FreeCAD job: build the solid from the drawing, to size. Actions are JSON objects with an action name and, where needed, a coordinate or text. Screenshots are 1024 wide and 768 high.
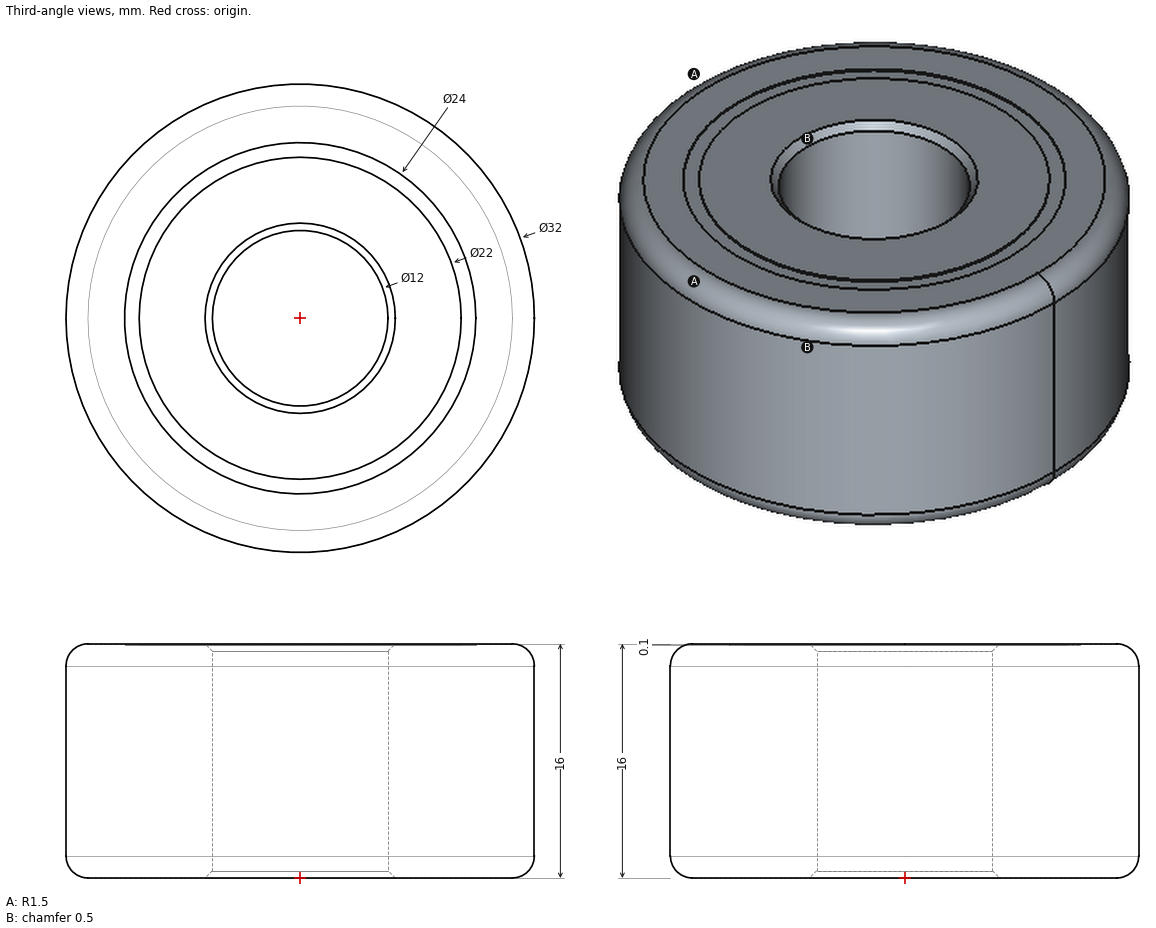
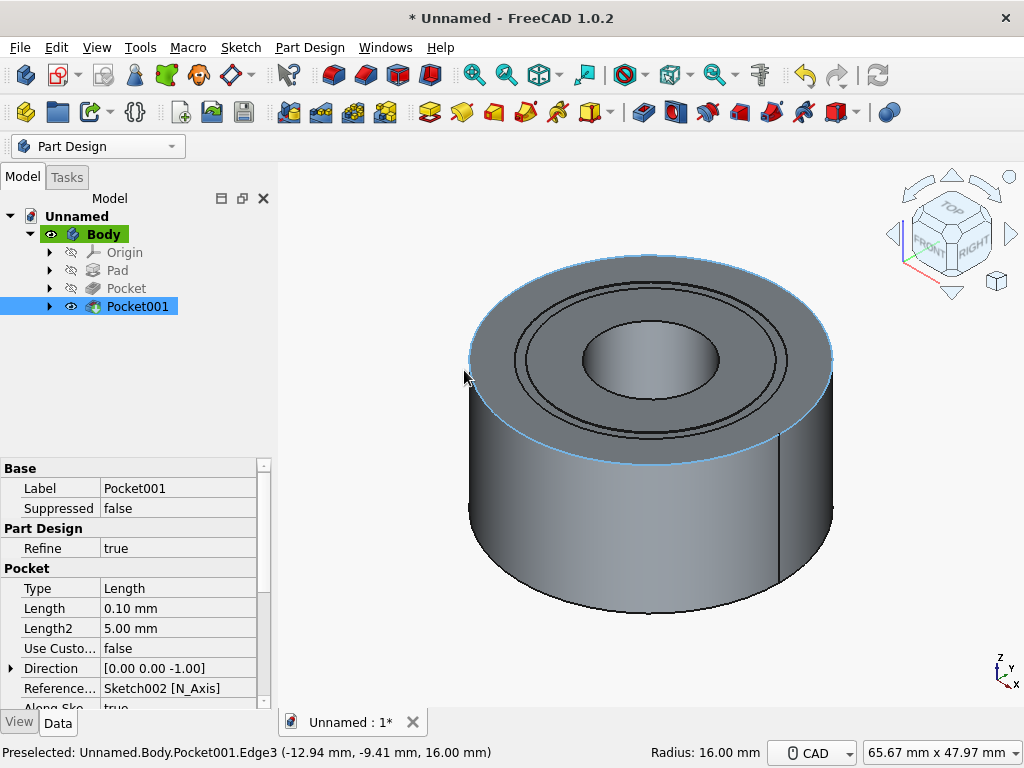
{"action": "key", "text": "2"}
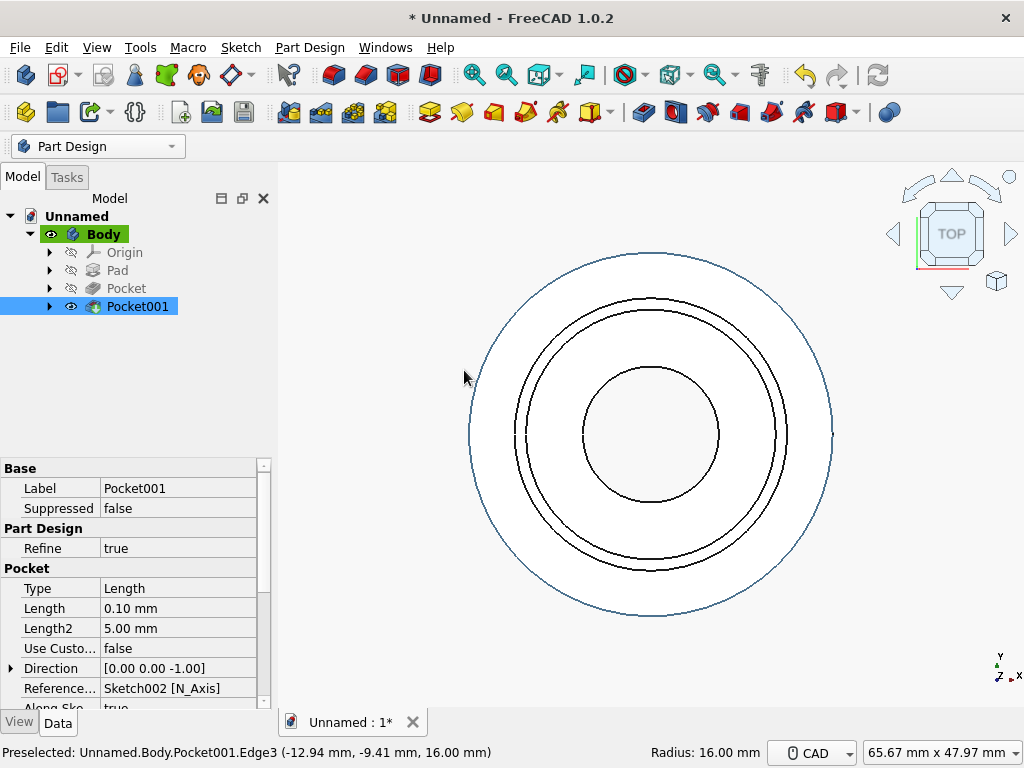
{"action": "key", "text": "1"}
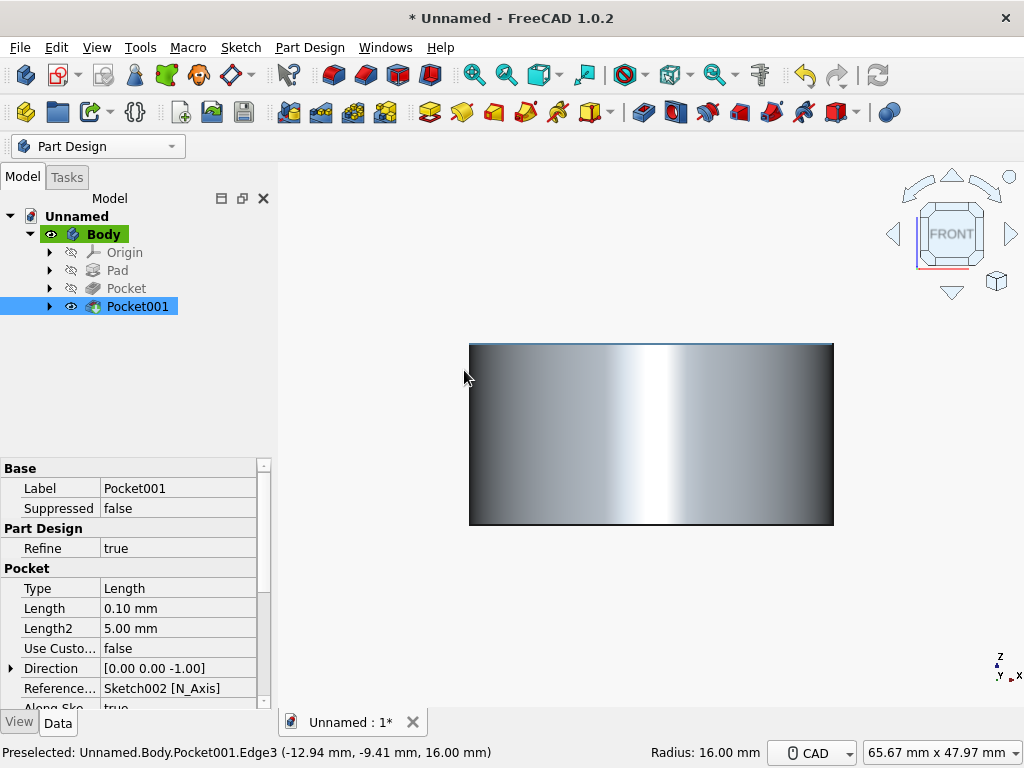
{"action": "left_click", "coordinate": [504, 524], "text": "ctrl"}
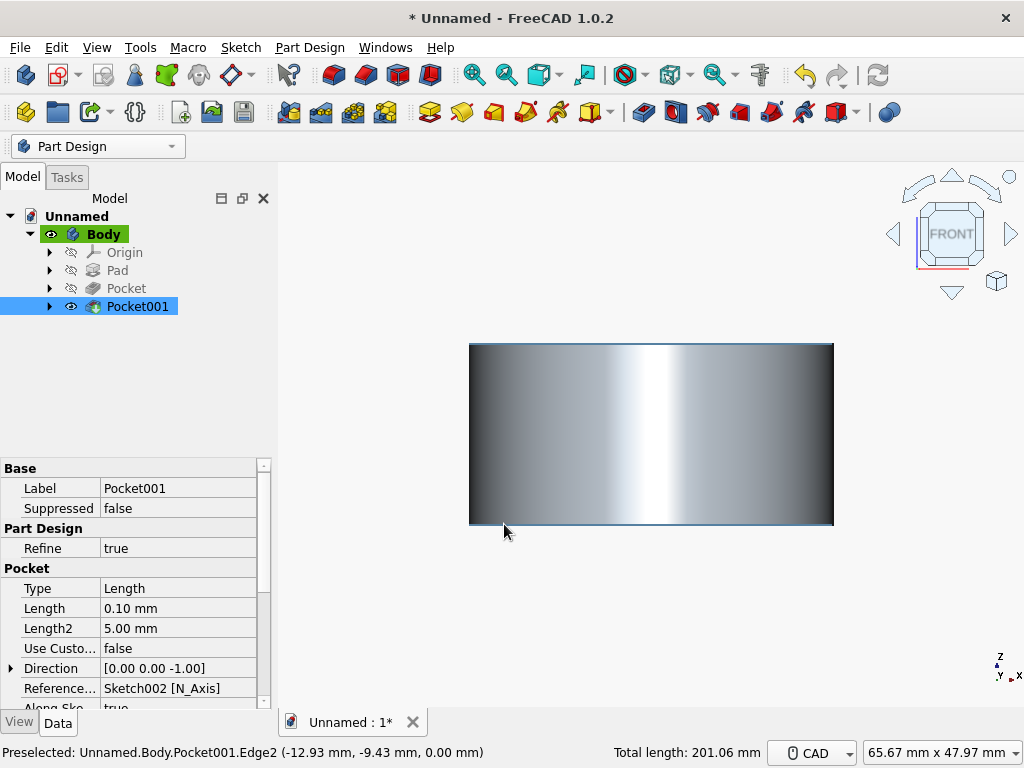
{"action": "left_click", "coordinate": [334, 76]}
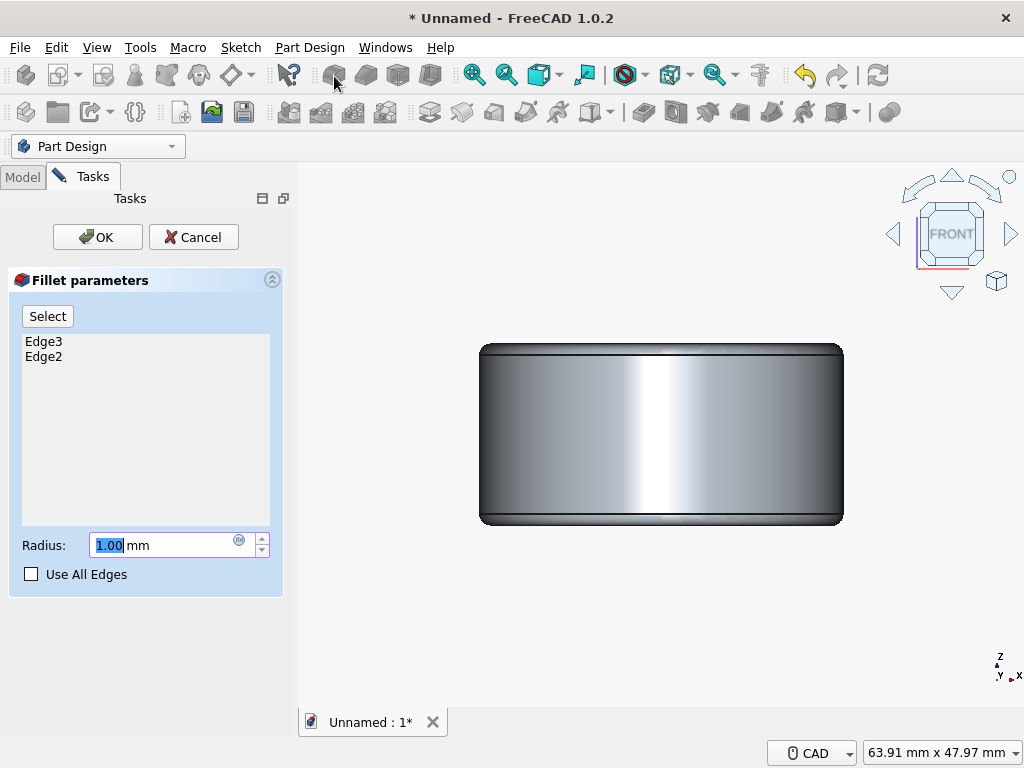
{"action": "type", "text": "1.5"}
{"action": "key", "text": "Tab"}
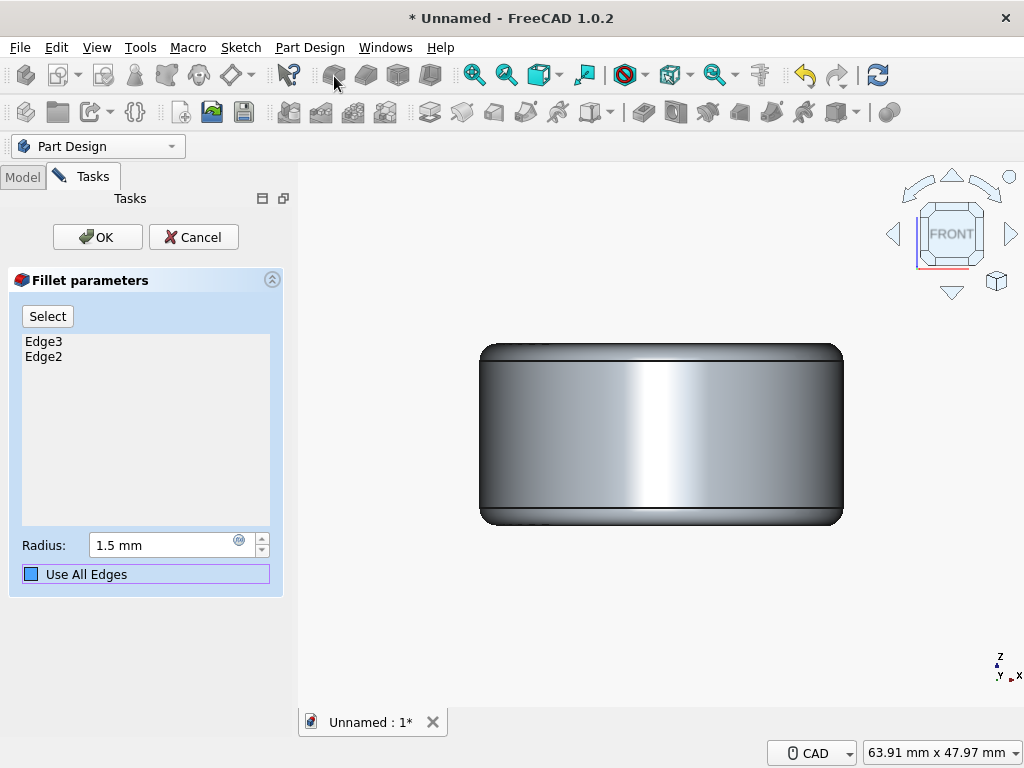
{"action": "left_click", "coordinate": [98, 237]}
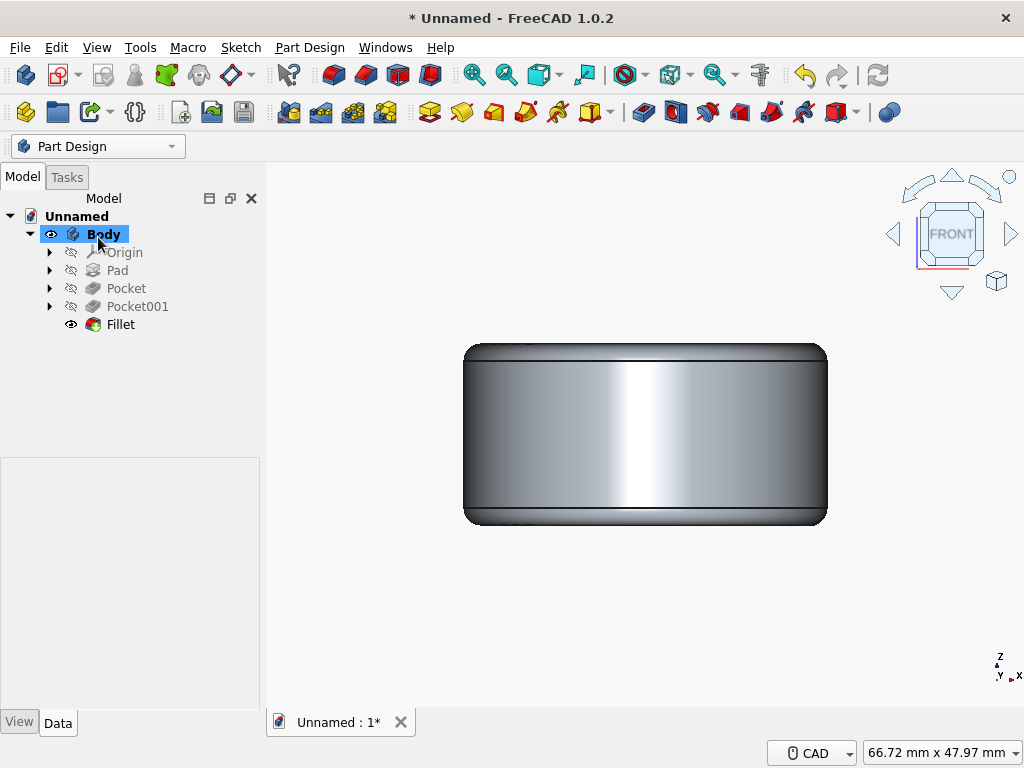
{"action": "key", "text": "0"}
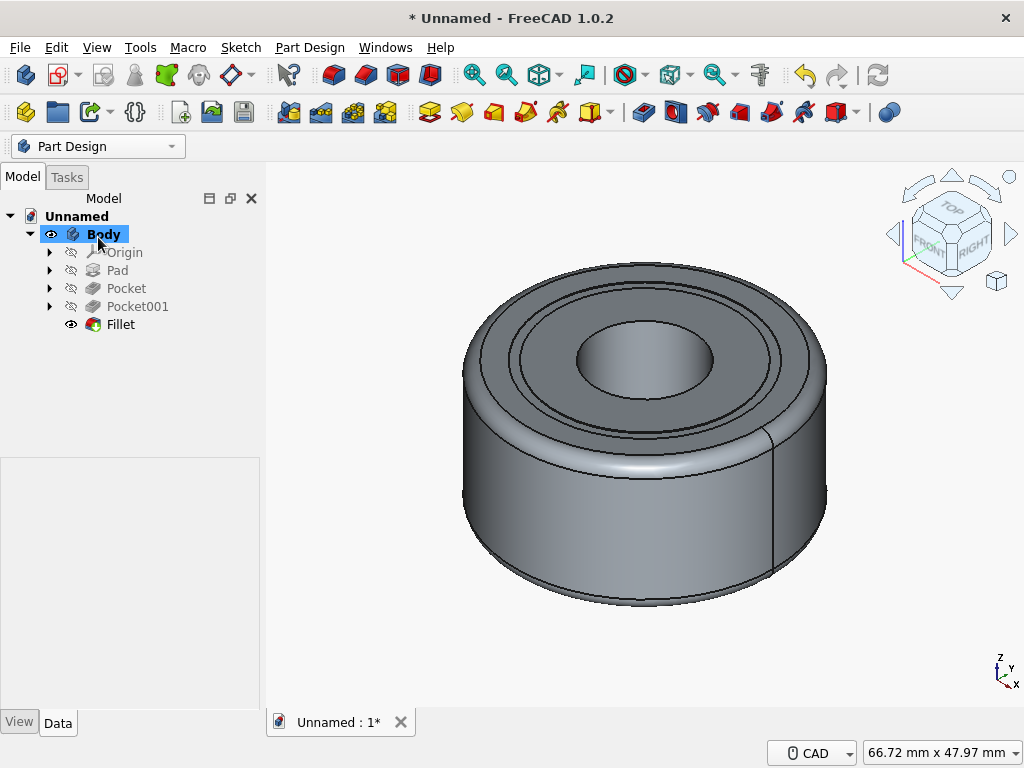
{"action": "left_click", "coordinate": [597, 331]}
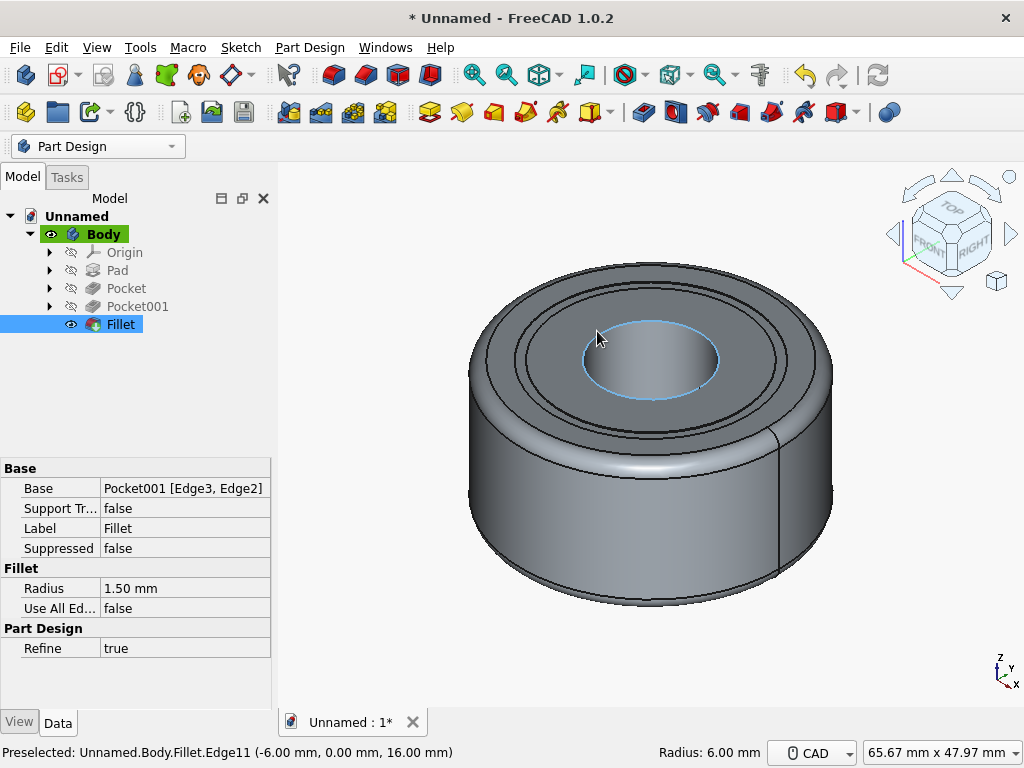
{"action": "key", "text": "2"}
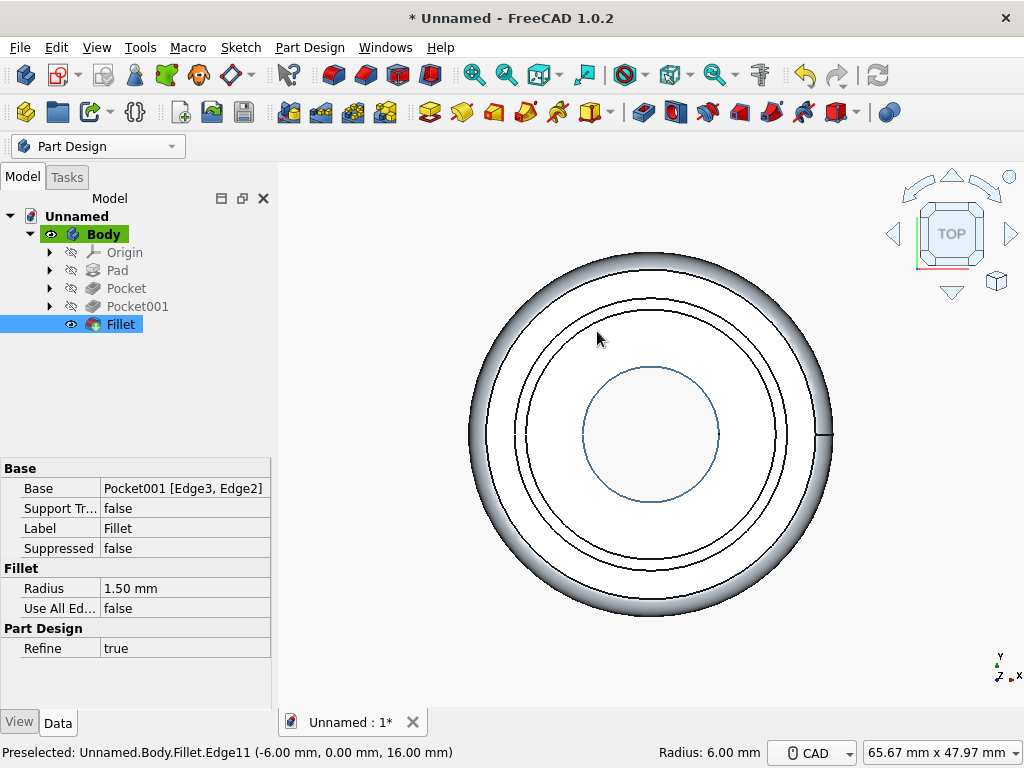
{"action": "key", "text": "1"}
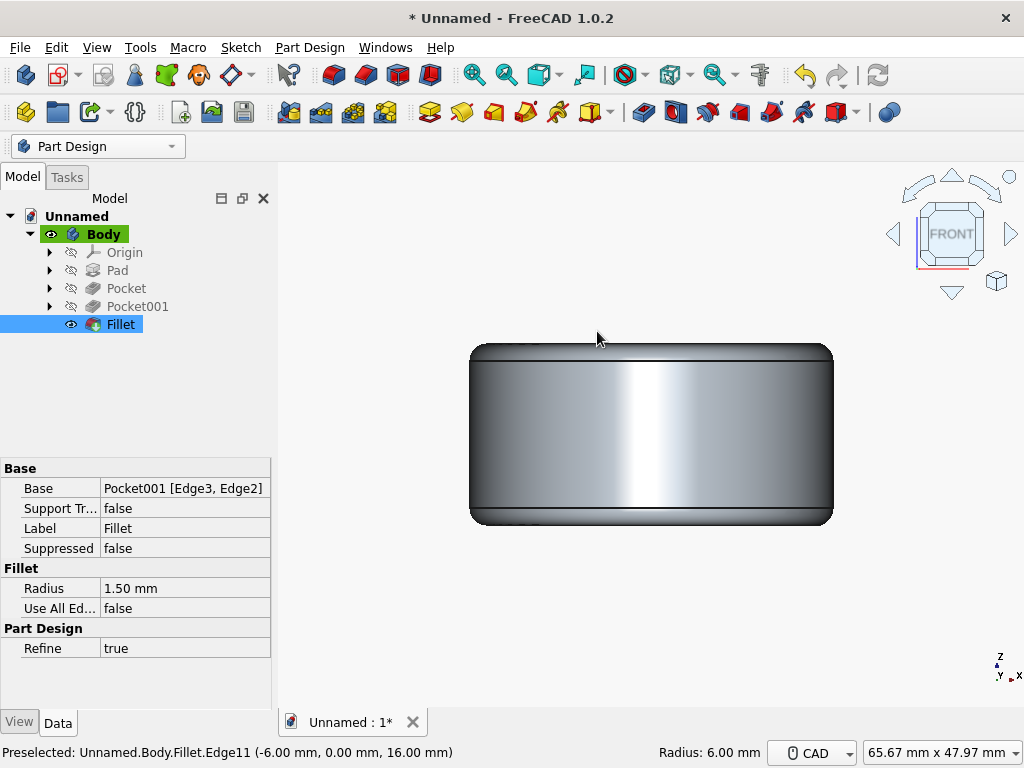
{"action": "key", "text": "3"}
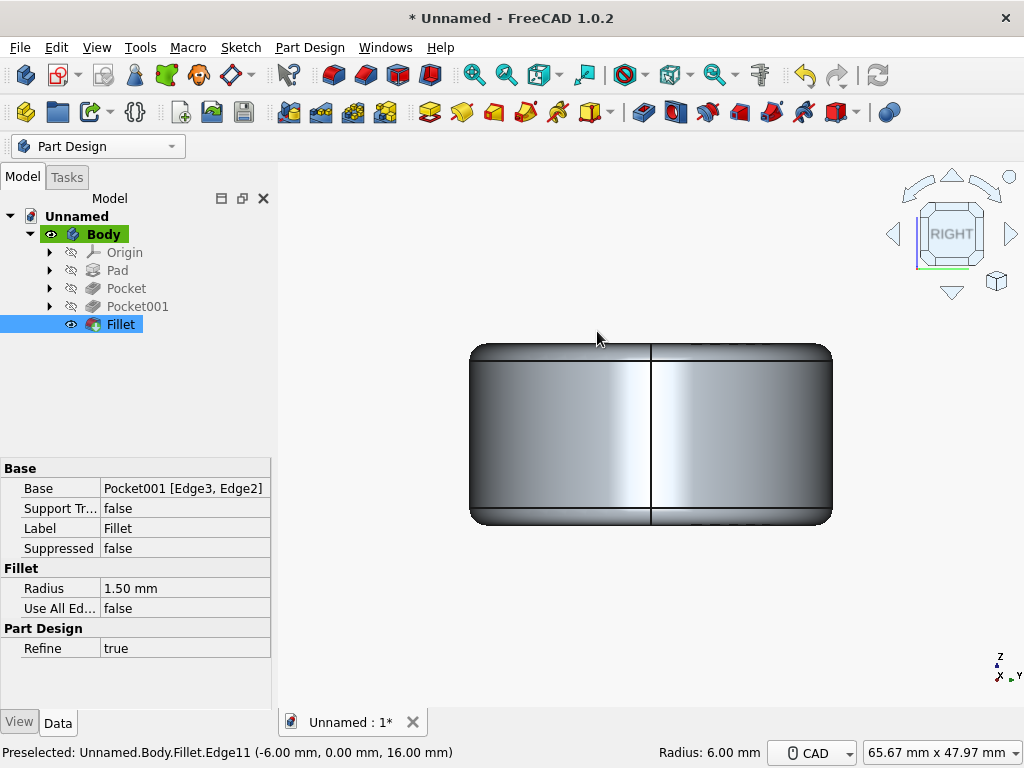
{"action": "key", "text": "5"}